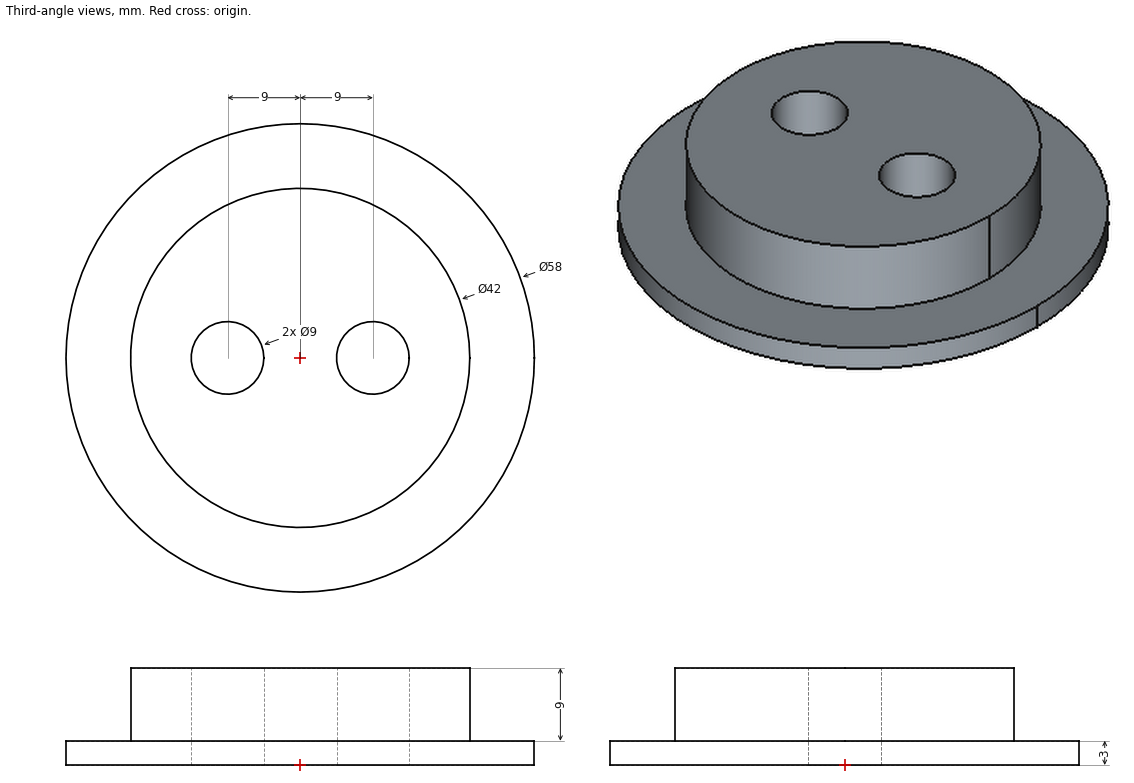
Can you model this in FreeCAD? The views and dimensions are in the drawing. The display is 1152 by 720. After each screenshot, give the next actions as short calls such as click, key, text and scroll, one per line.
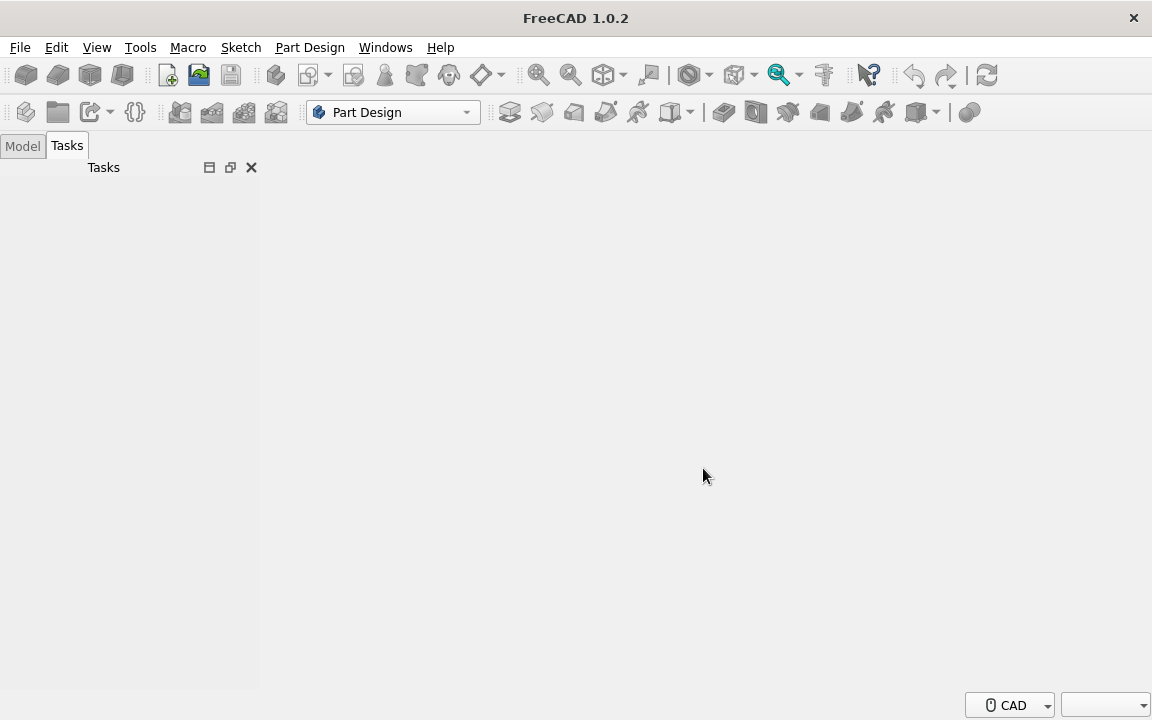
click(168, 76)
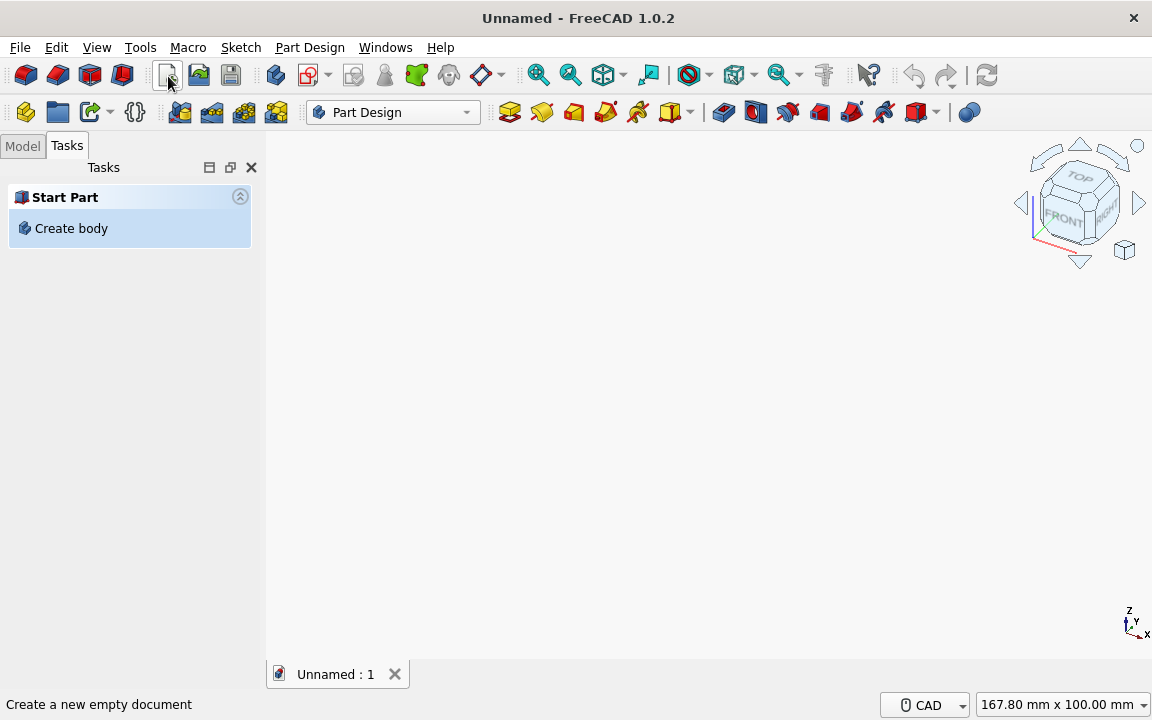
click(308, 76)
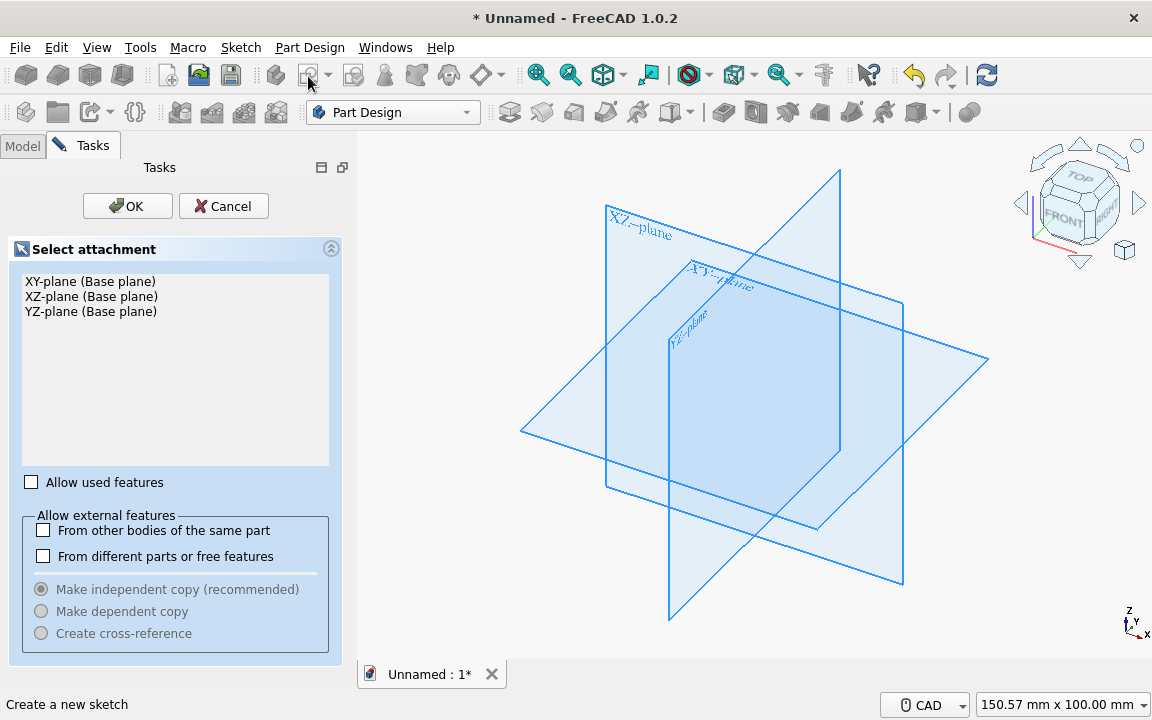
click(82, 282)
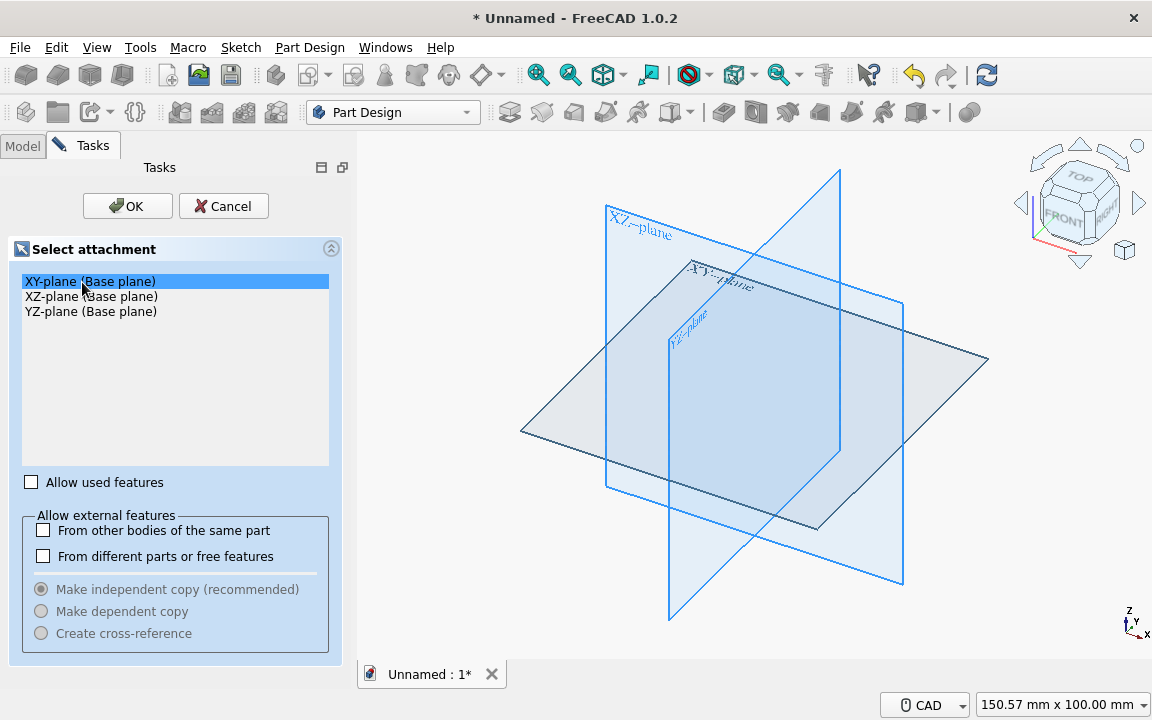
click(128, 206)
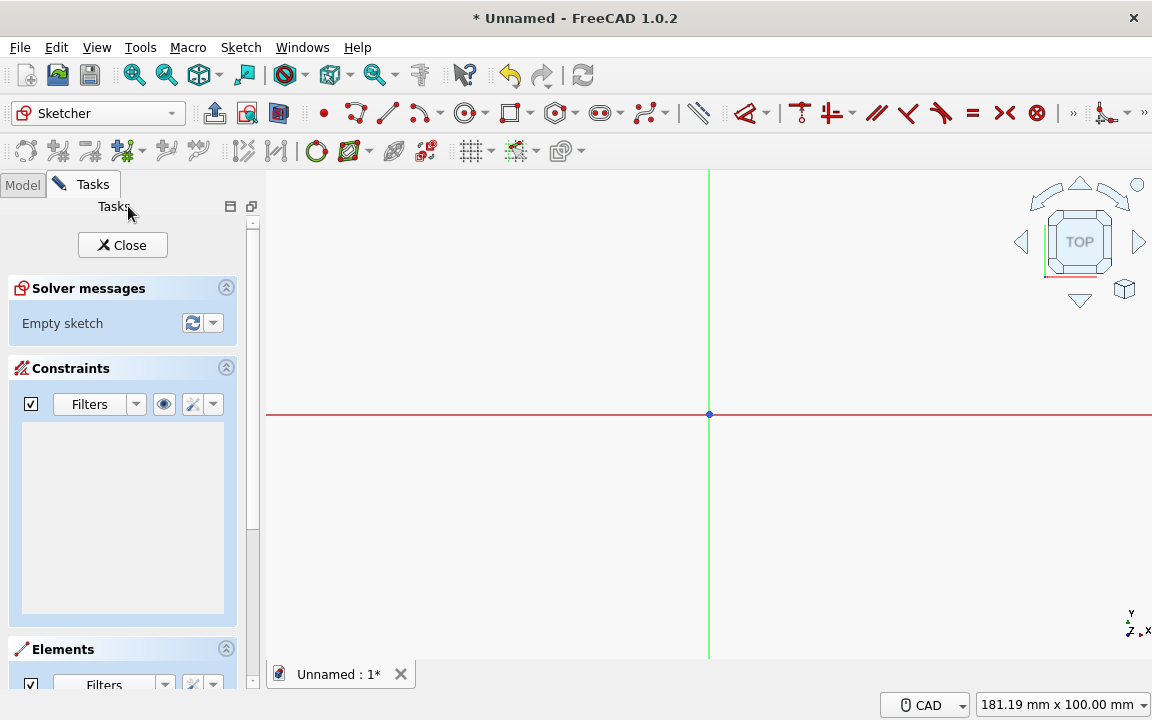
click(466, 114)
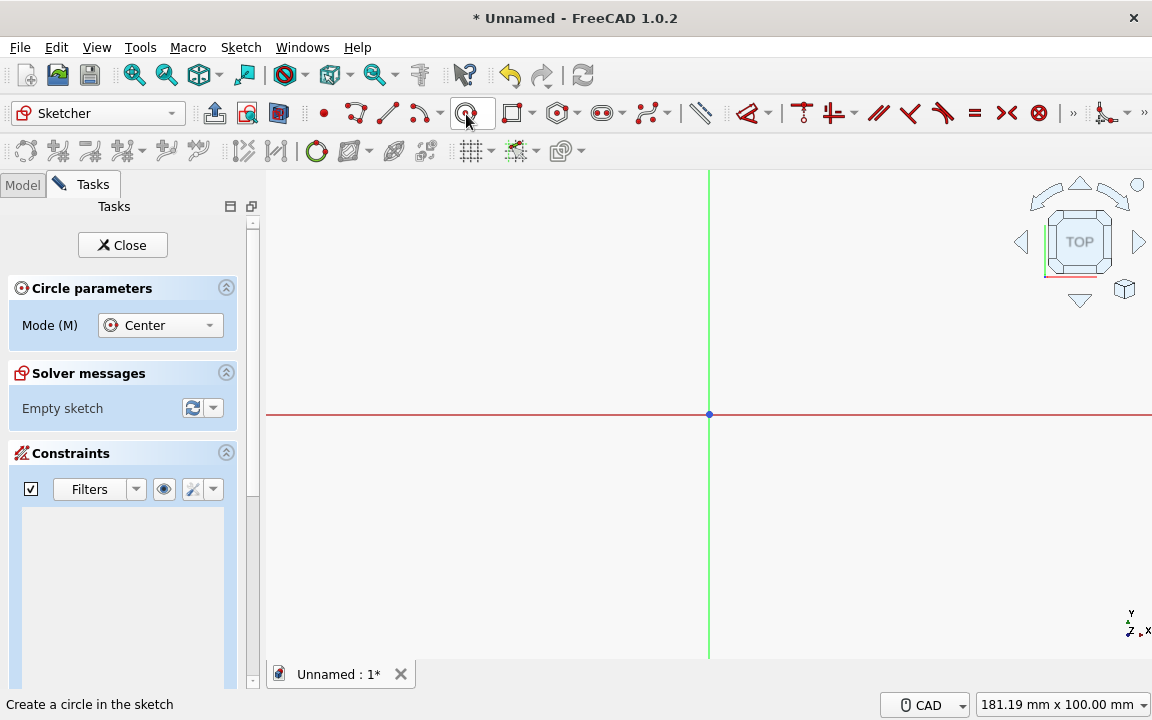
click(709, 414)
move(809, 314)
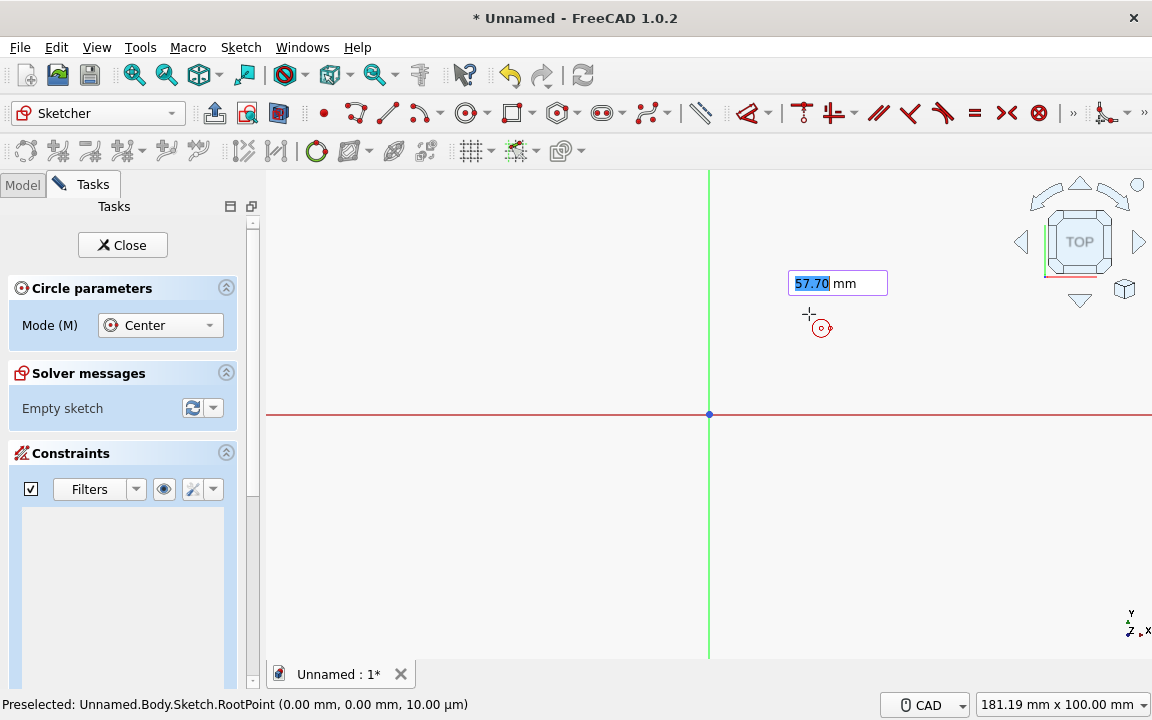
text(58)
key(Return)
key(Escape)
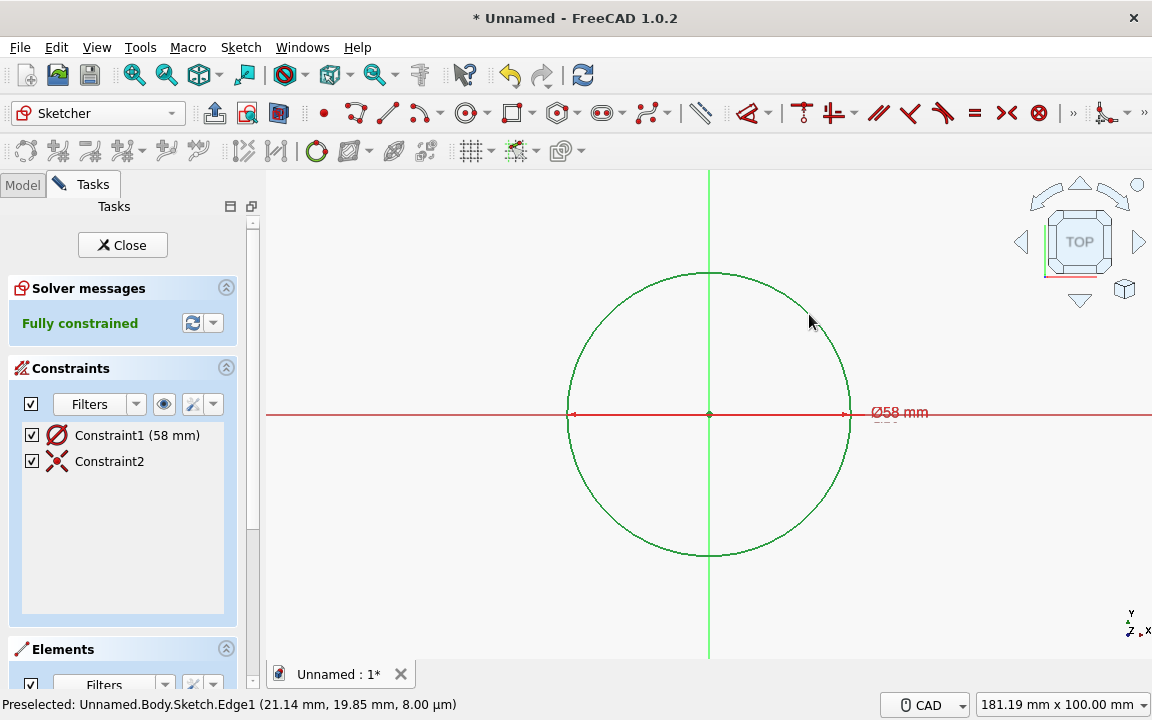
click(123, 245)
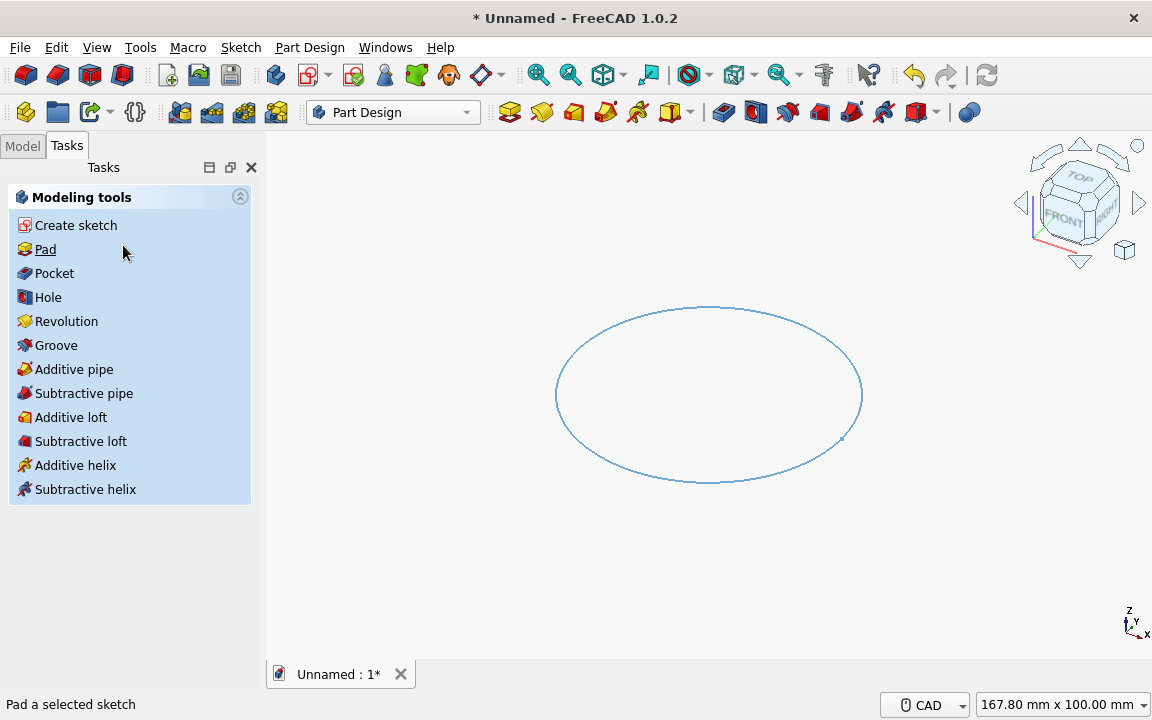
click(510, 112)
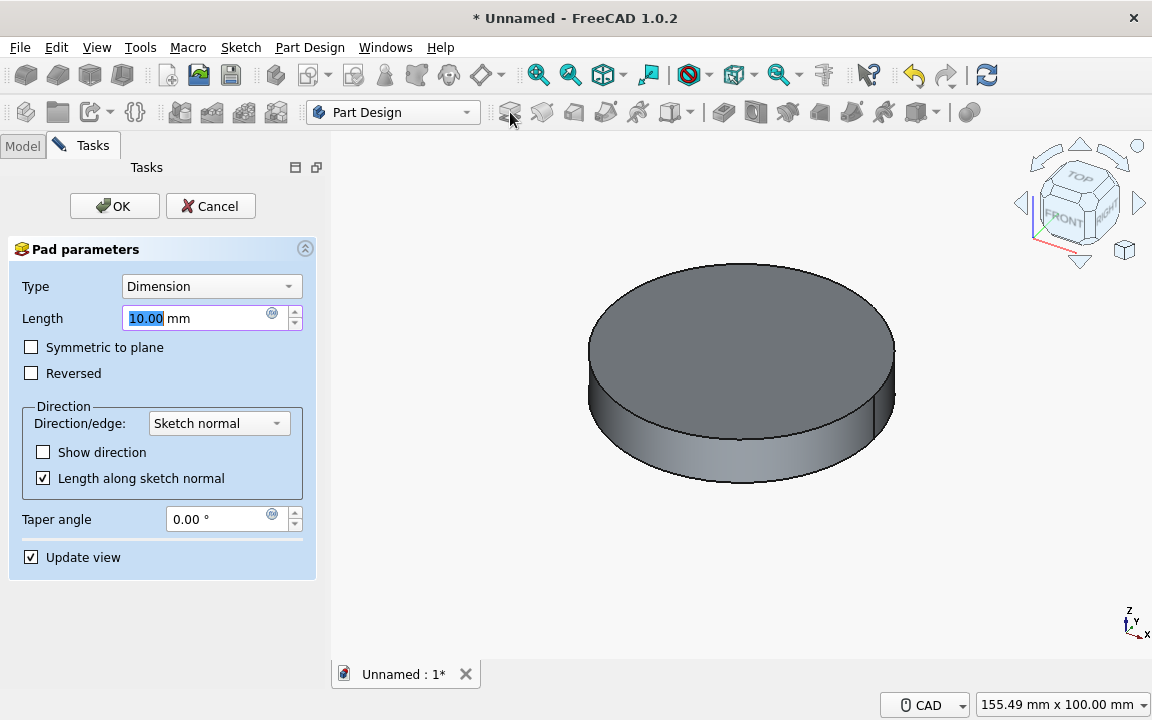
text(3)
key(Tab)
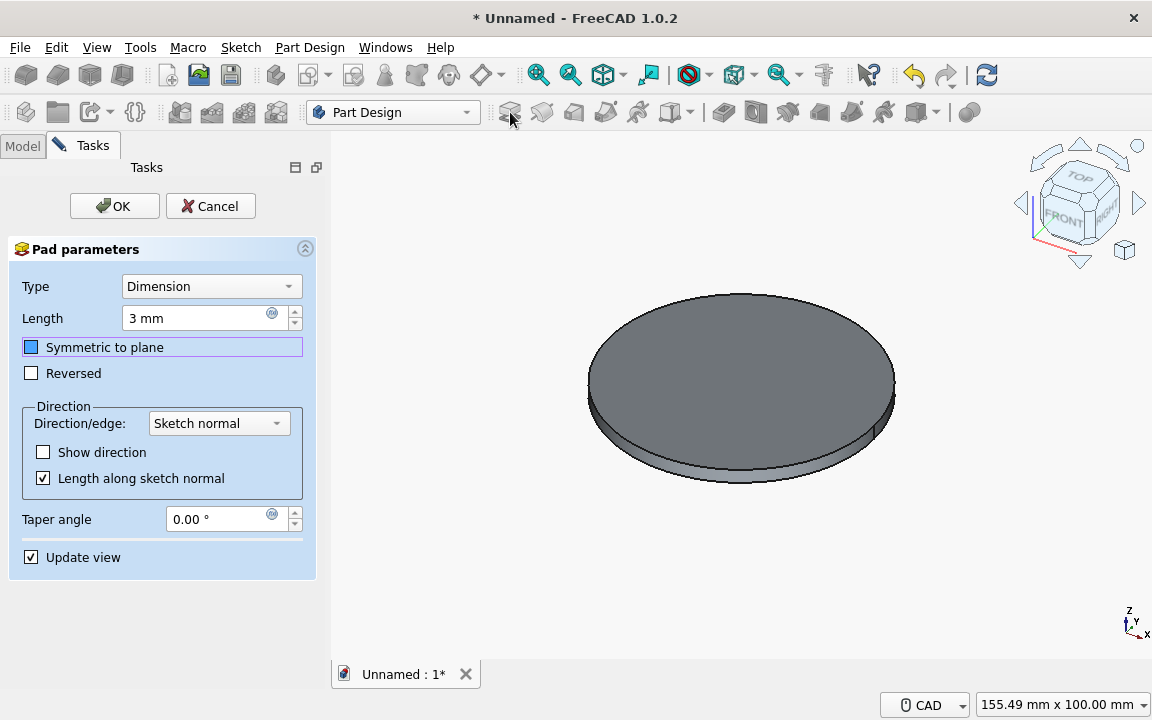
click(115, 206)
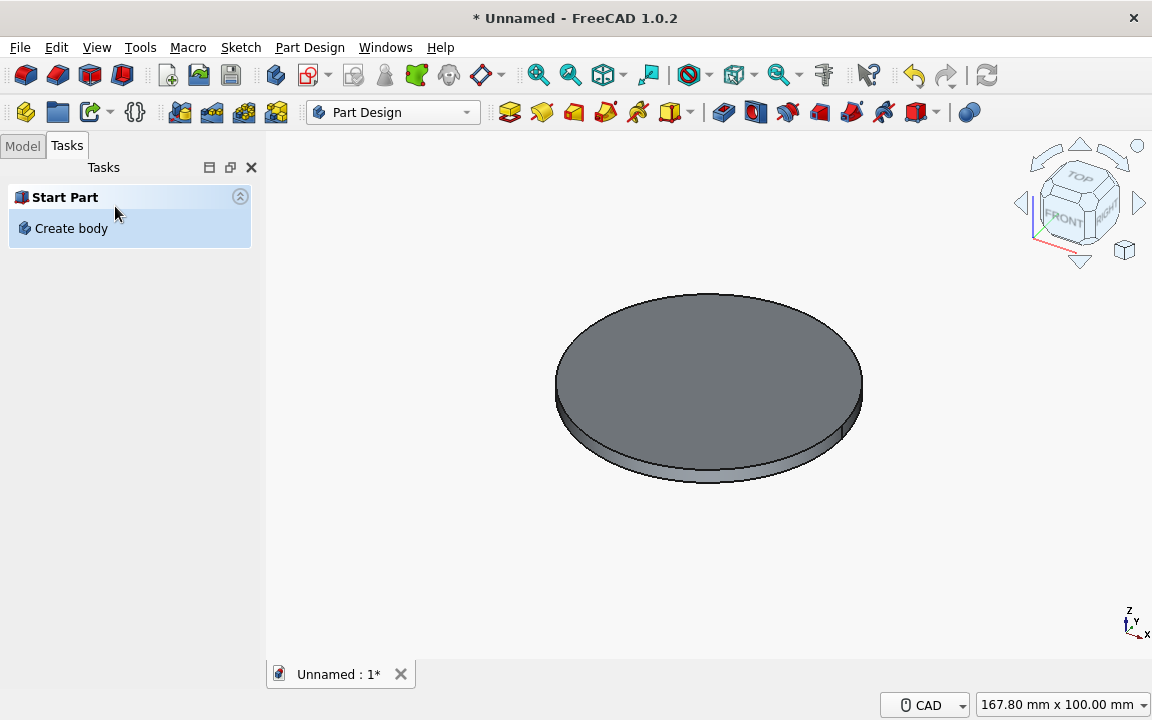
click(709, 381)